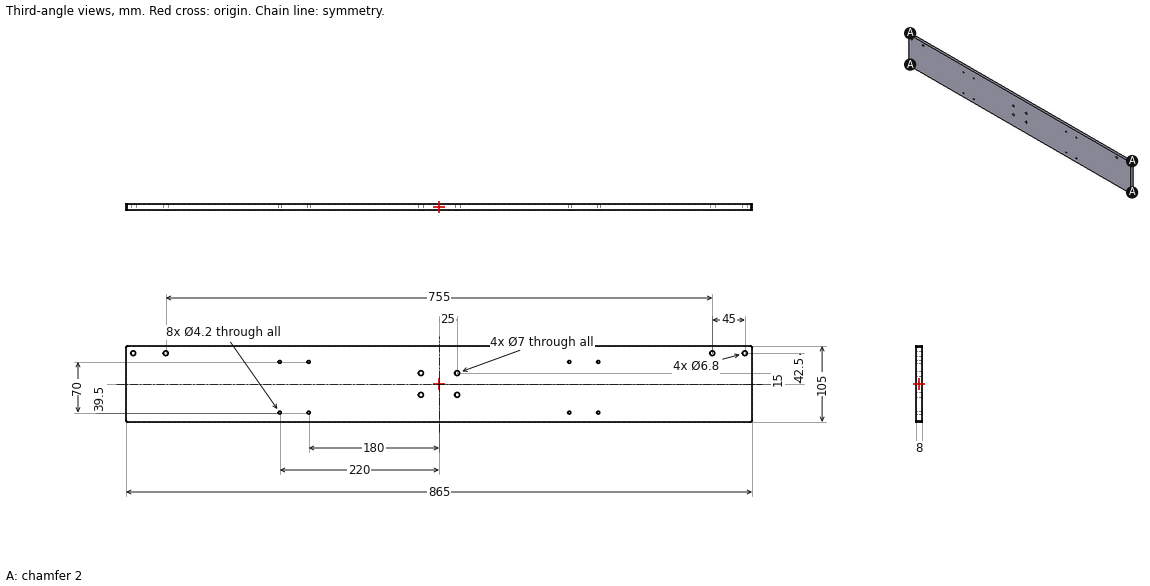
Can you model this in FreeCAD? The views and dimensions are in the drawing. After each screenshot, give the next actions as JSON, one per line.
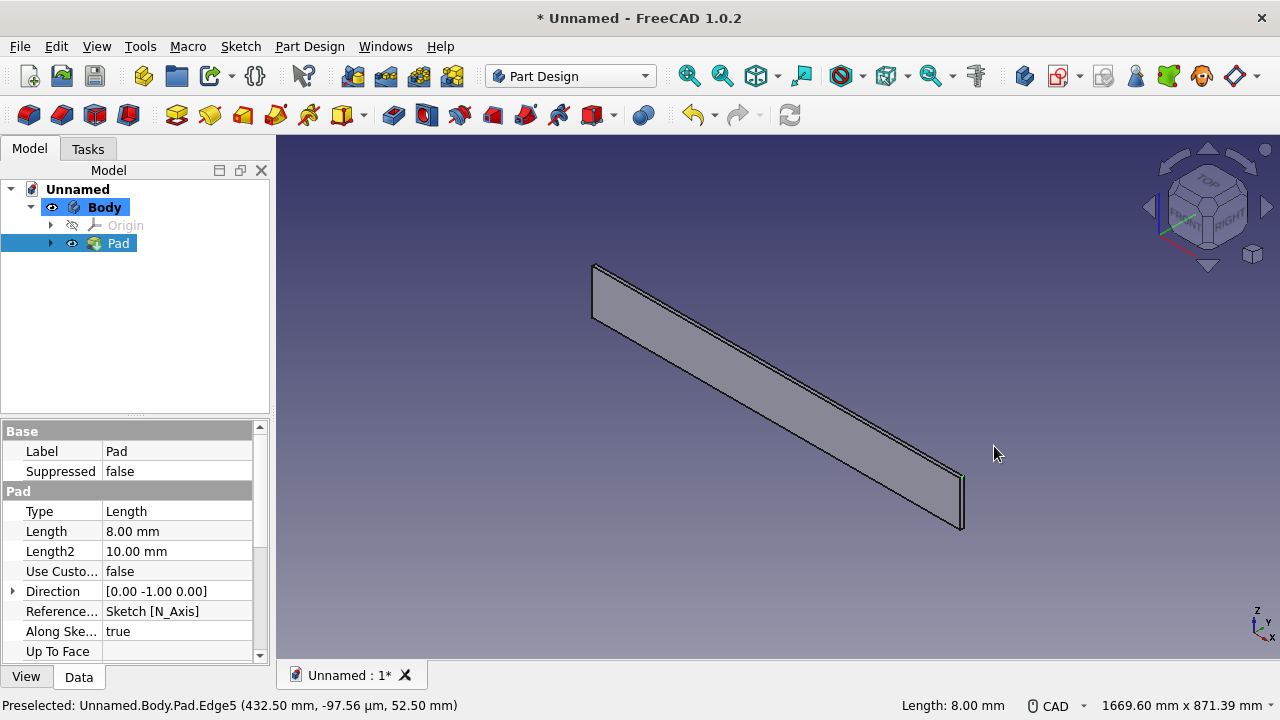
{"action": "scroll", "coordinate": [594, 264], "scroll_direction": "up", "scroll_amount": 11}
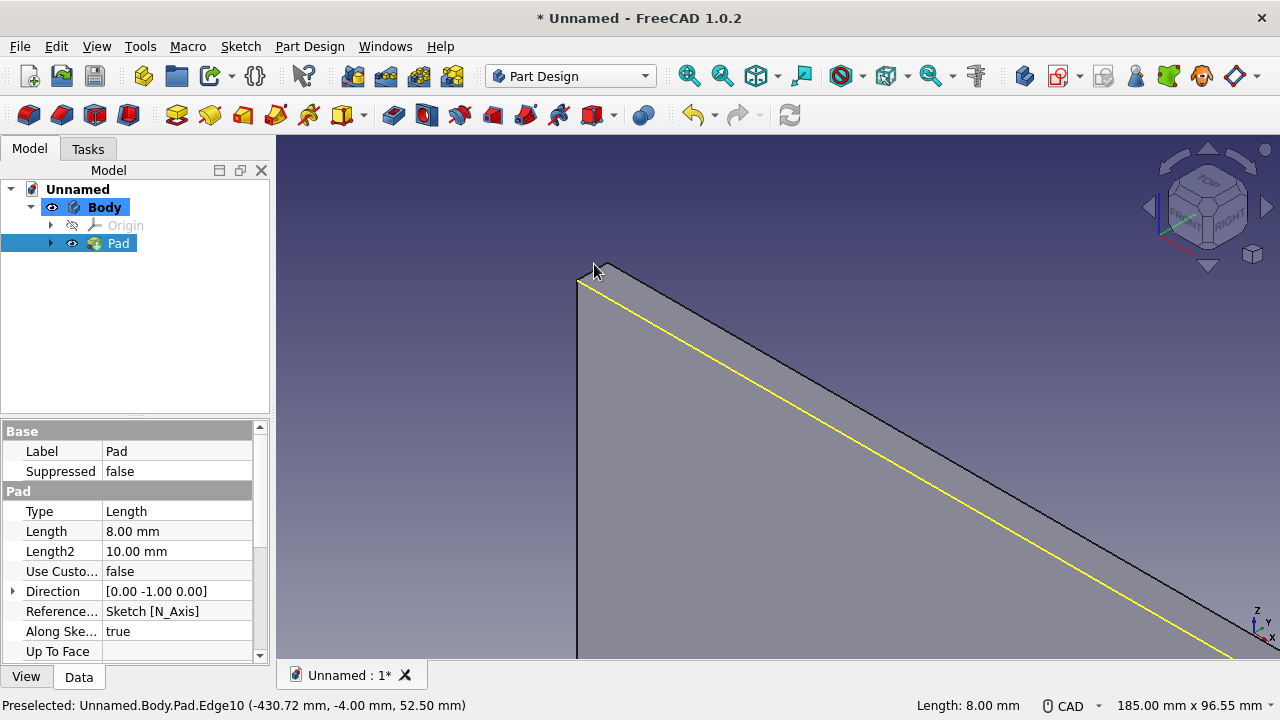
{"action": "key", "text": "v f"}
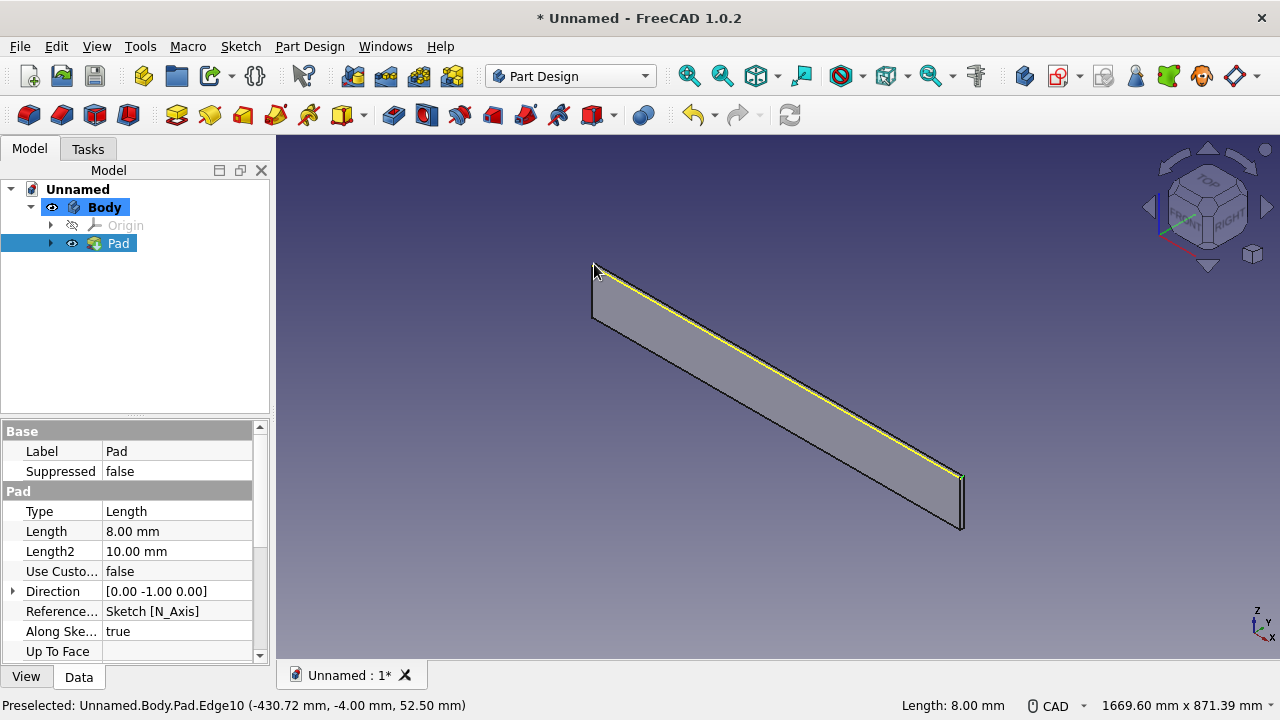
{"action": "key", "text": "2"}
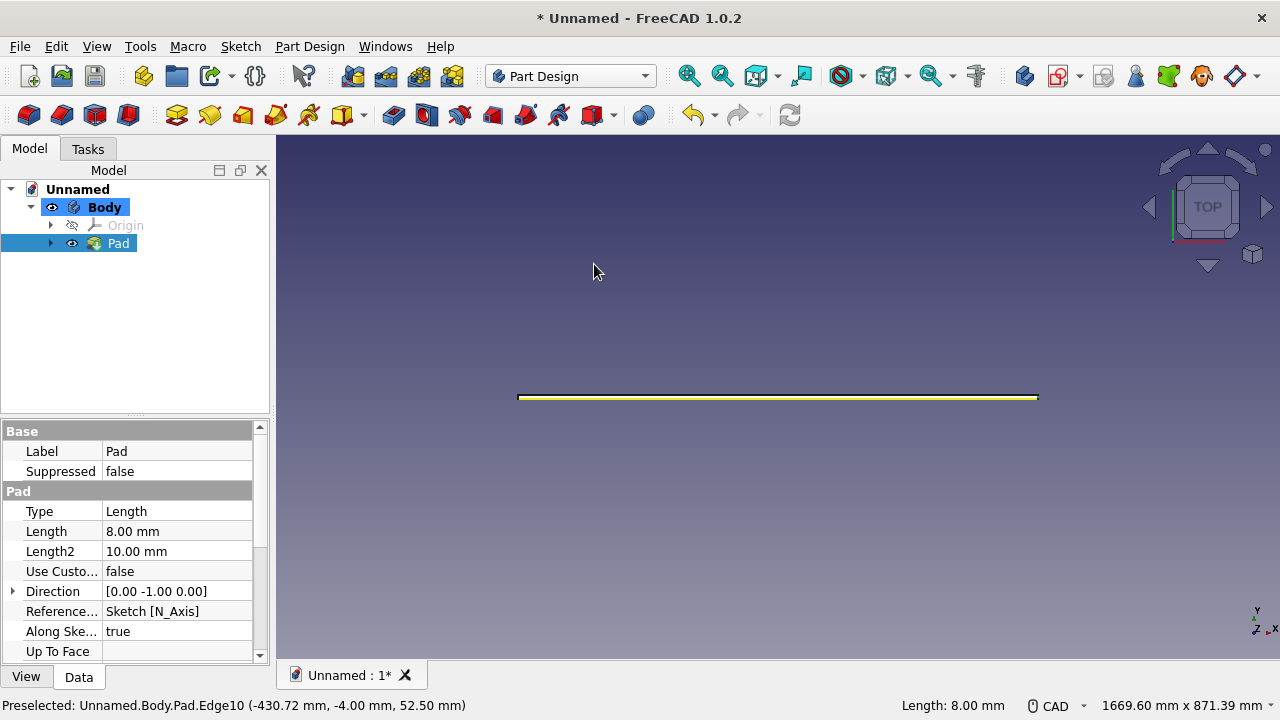
{"action": "scroll", "coordinate": [518, 396], "scroll_direction": "up", "scroll_amount": 11}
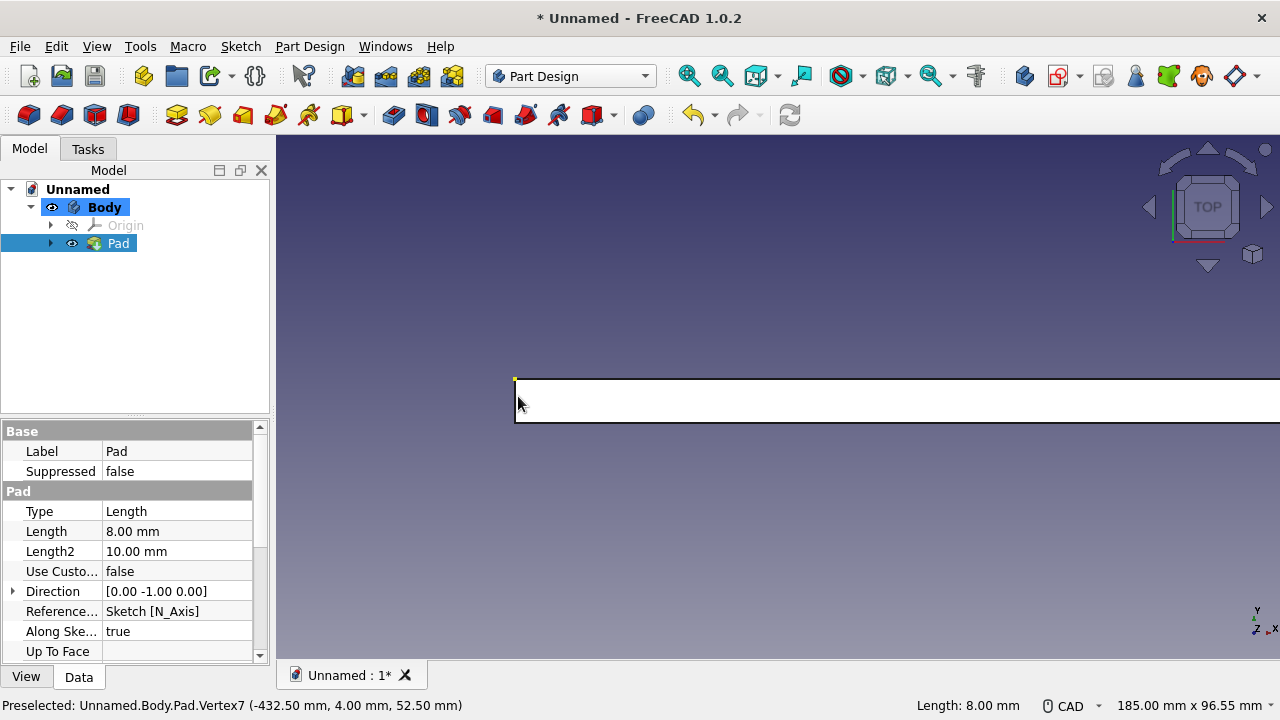
{"action": "left_click", "coordinate": [515, 400], "text": "ctrl"}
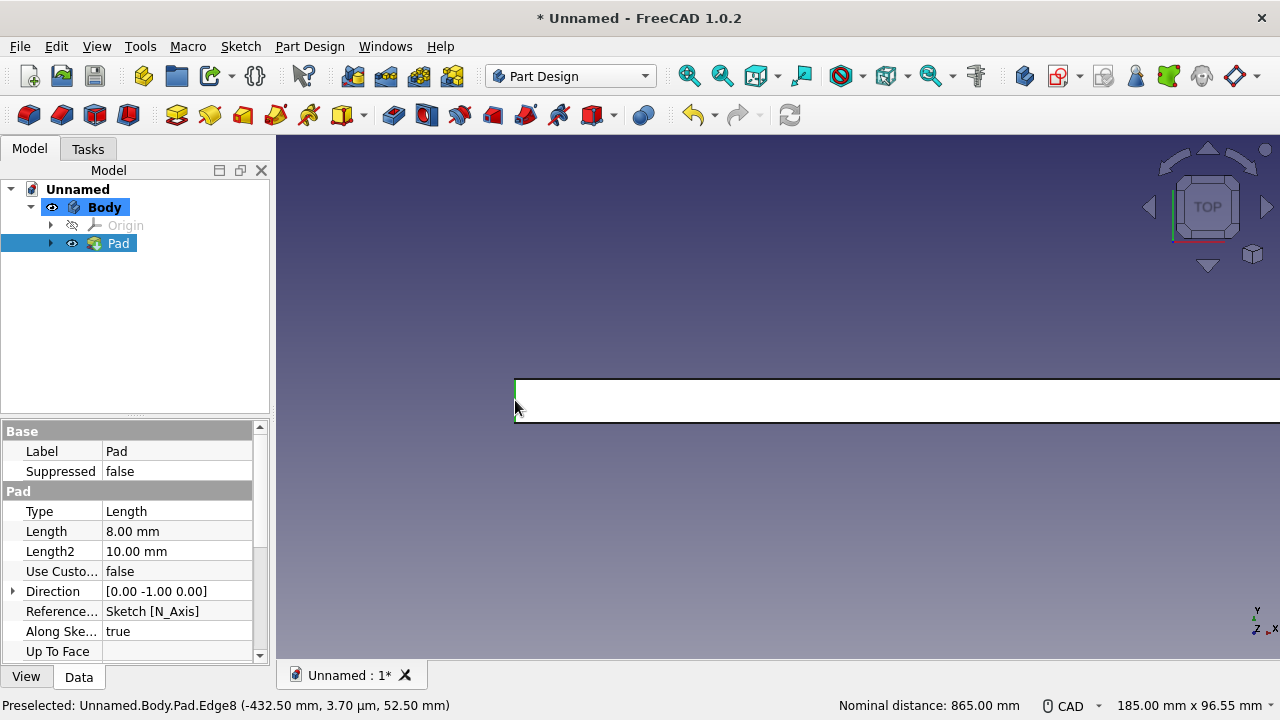
{"action": "key", "text": "v f"}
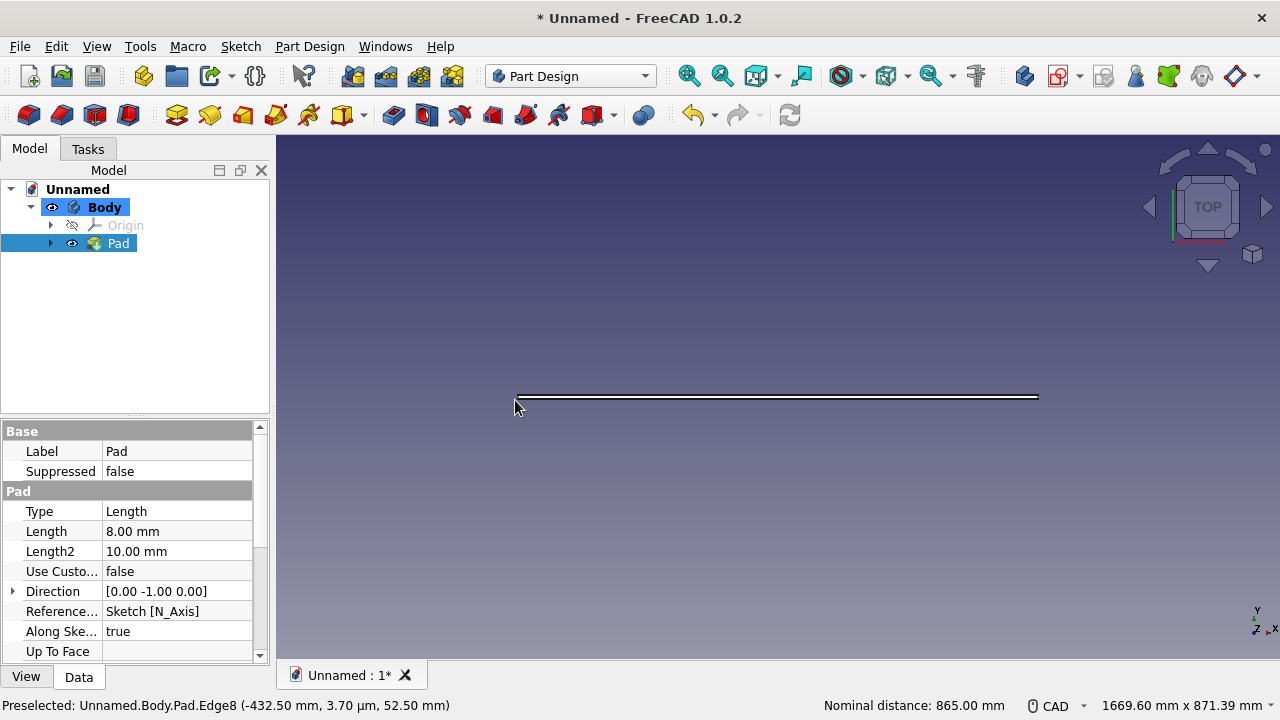
{"action": "key", "text": "1"}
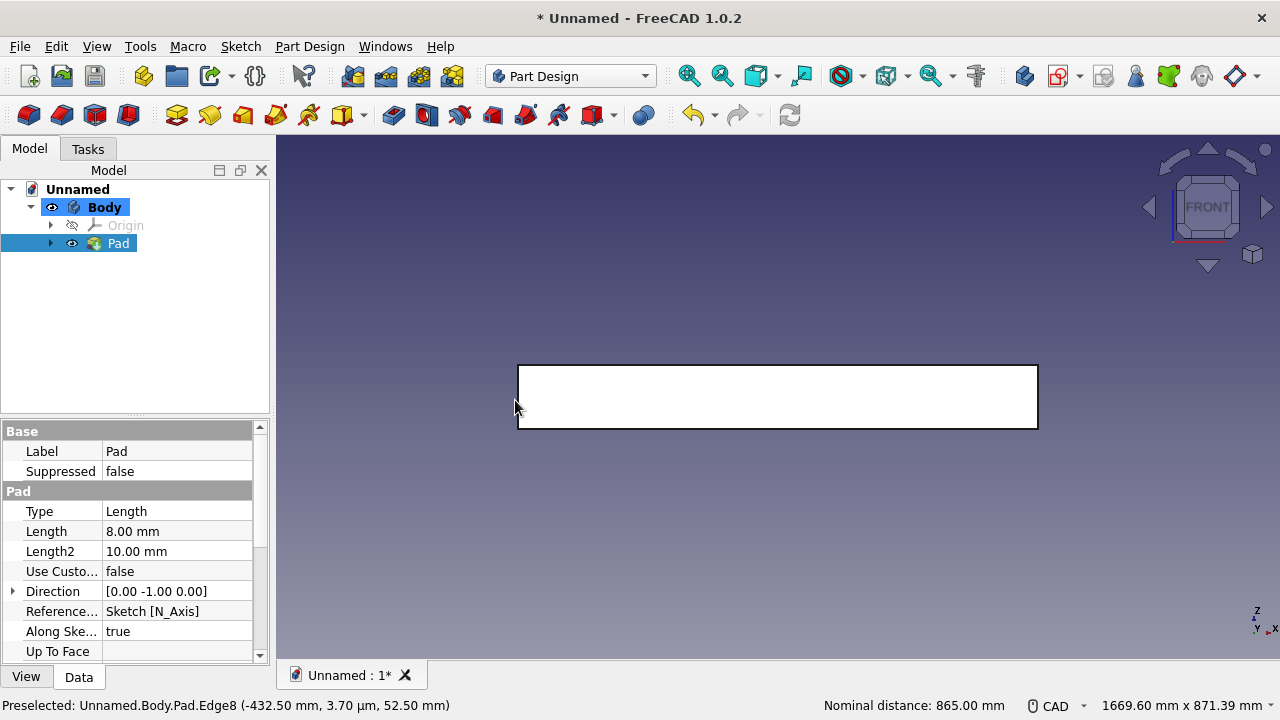
{"action": "scroll", "coordinate": [518, 428], "scroll_direction": "up", "scroll_amount": 11}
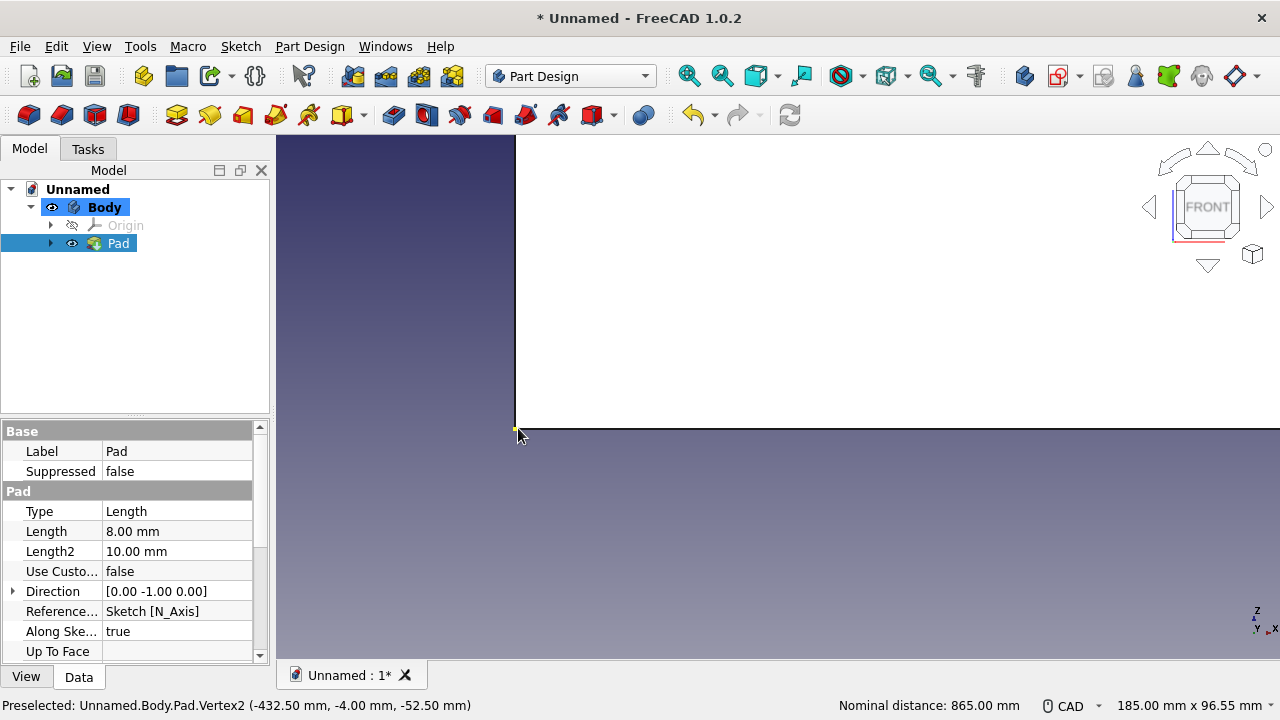
{"action": "left_click", "coordinate": [690, 76]}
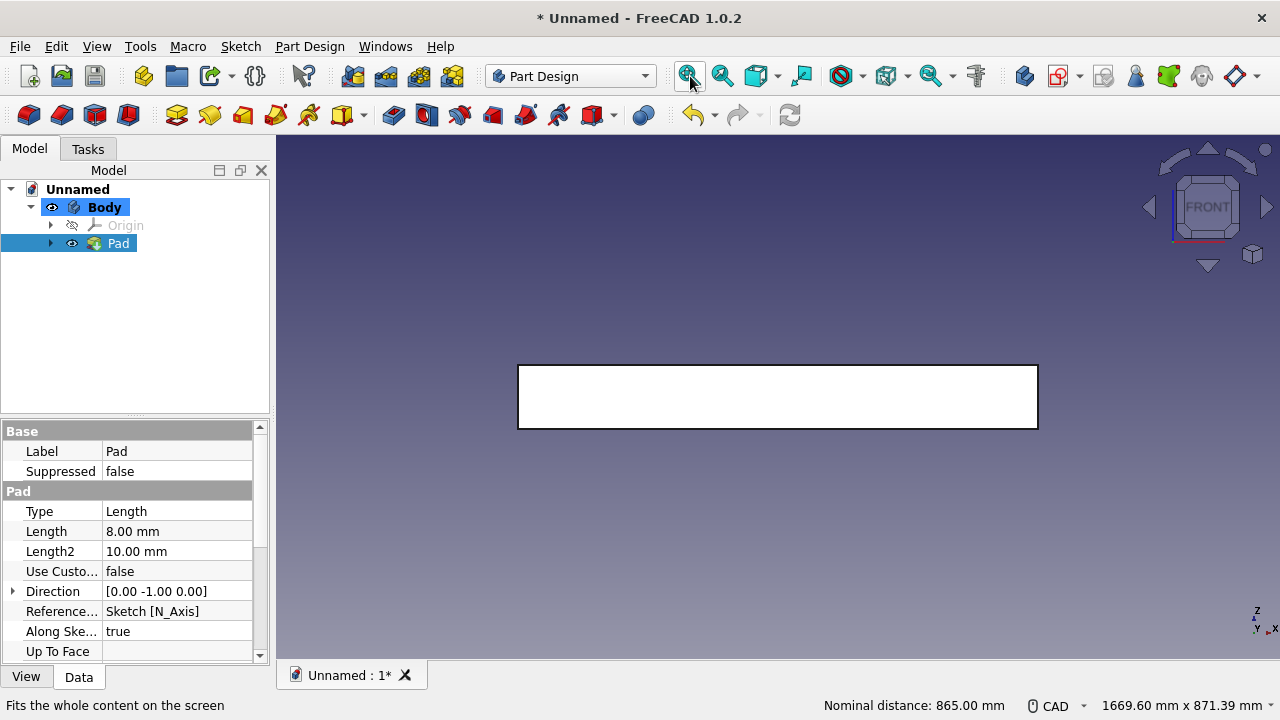
{"action": "key", "text": "3"}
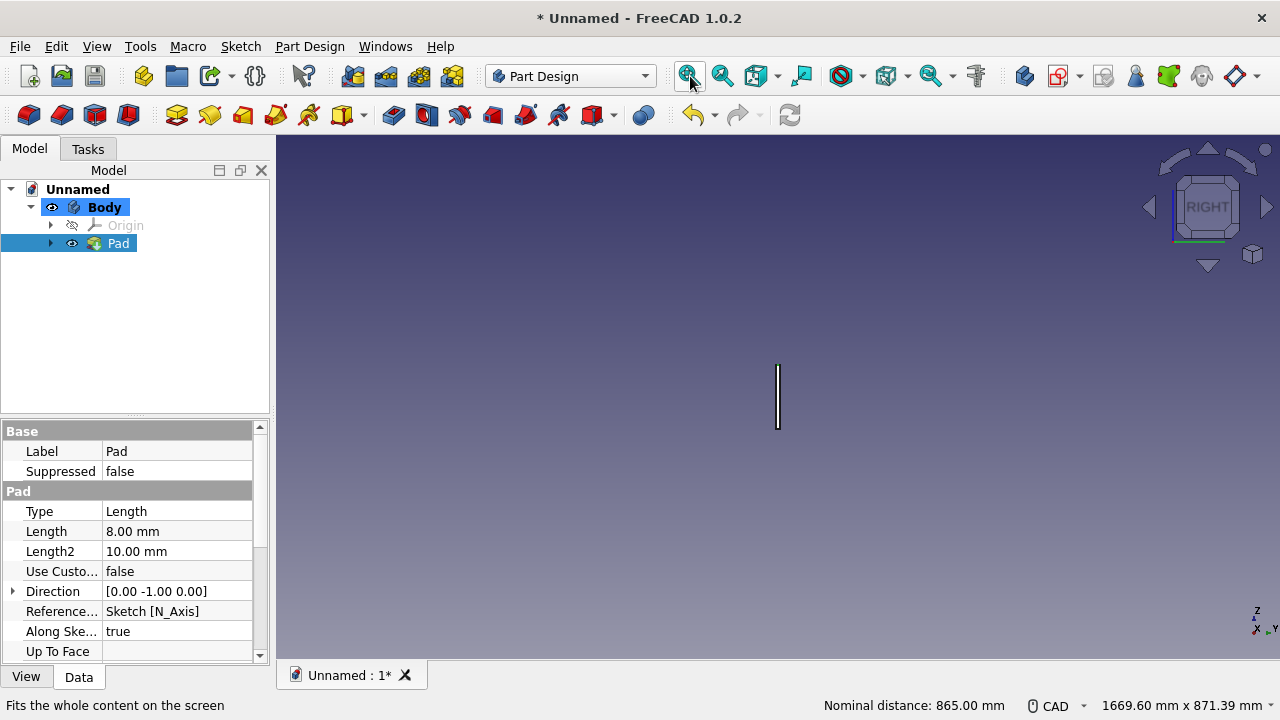
{"action": "key", "text": "v f"}